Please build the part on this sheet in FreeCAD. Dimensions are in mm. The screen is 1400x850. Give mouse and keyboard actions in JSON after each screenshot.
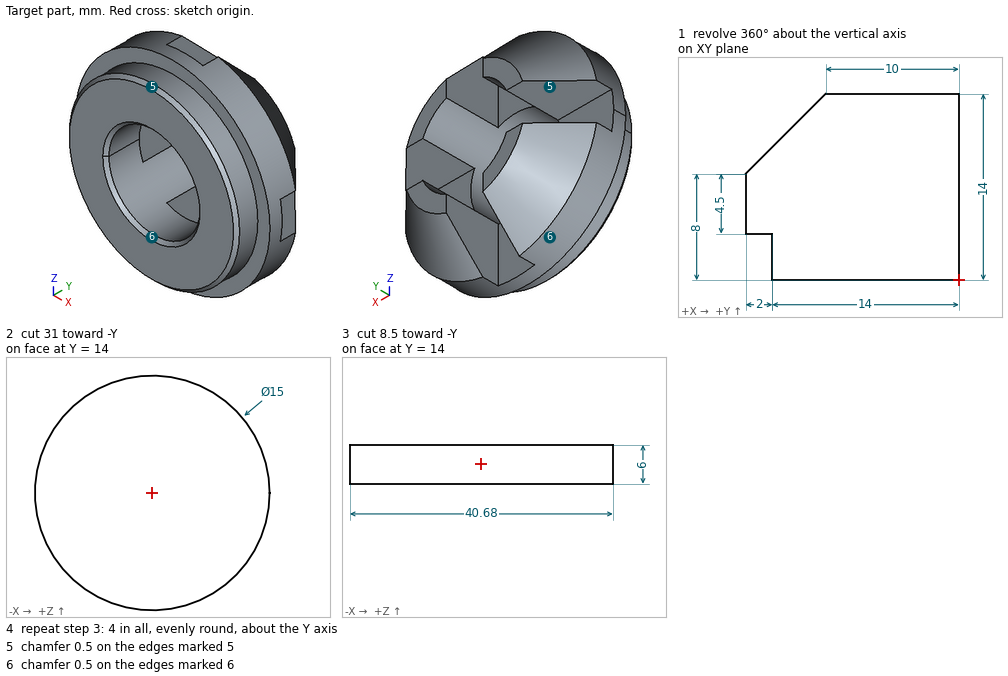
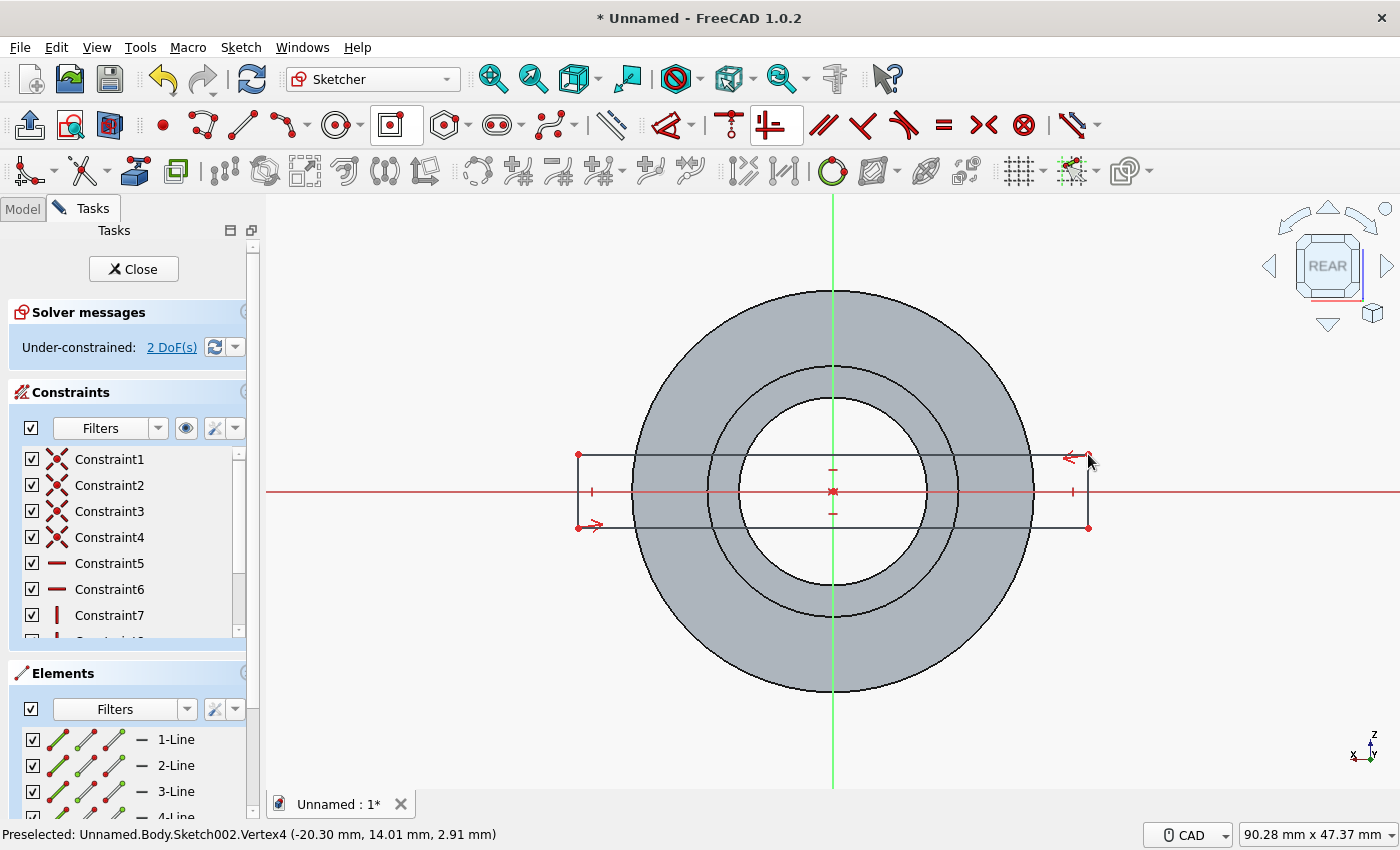
{"action": "left_click", "coordinate": [666, 126]}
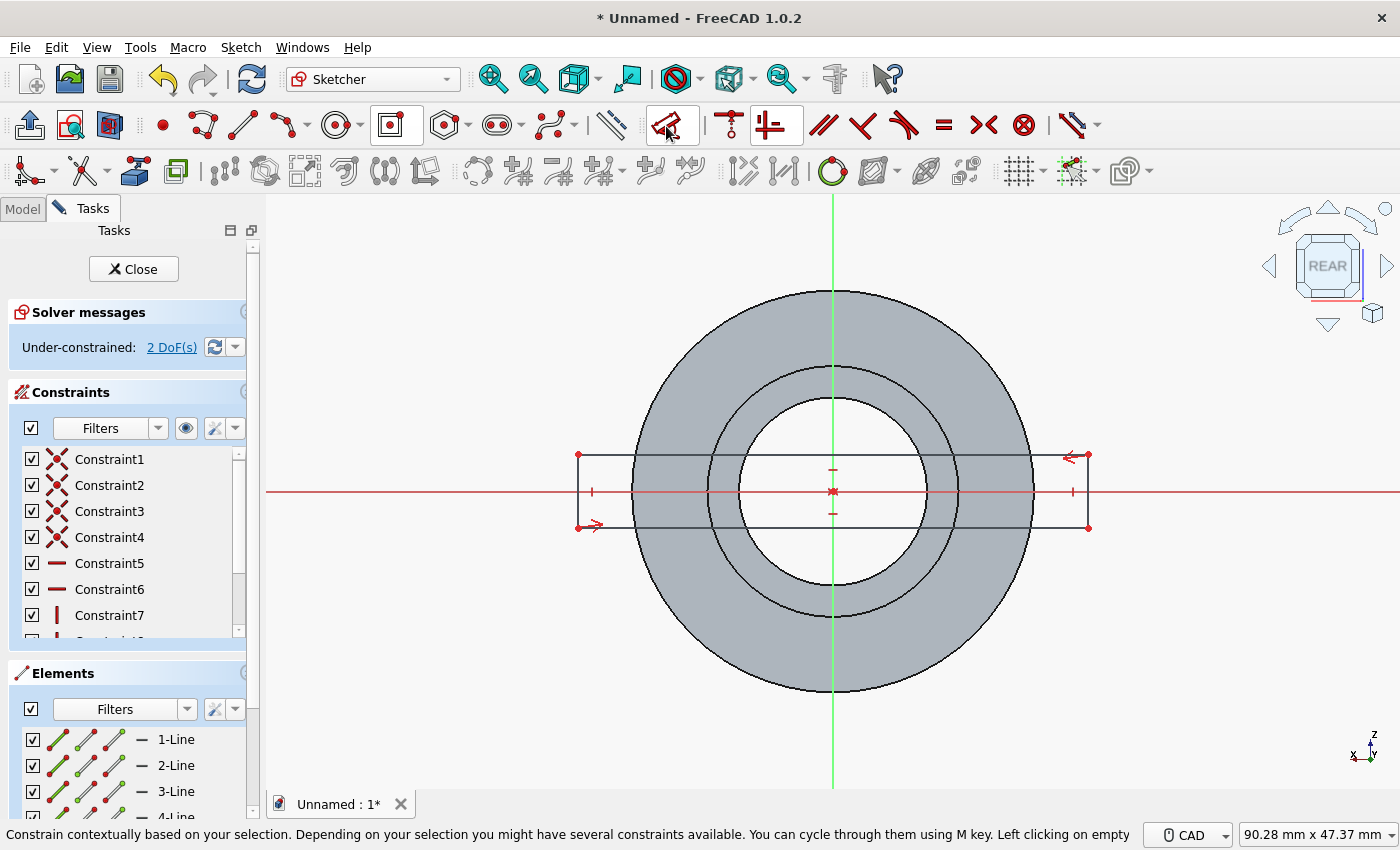
{"action": "left_click", "coordinate": [1088, 506]}
{"action": "left_click", "coordinate": [1122, 475]}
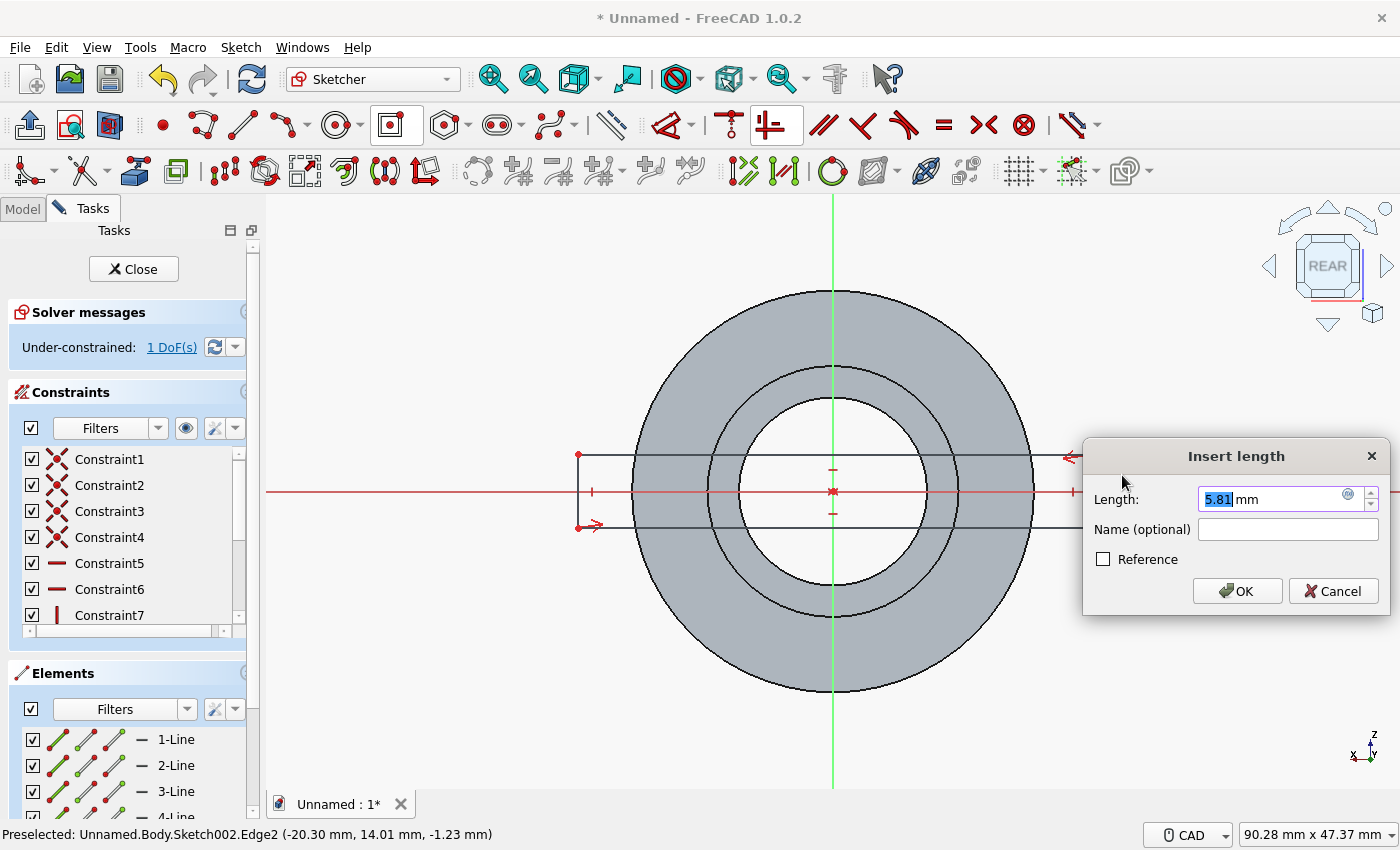
{"action": "type", "text": "6"}
{"action": "key", "text": "Return"}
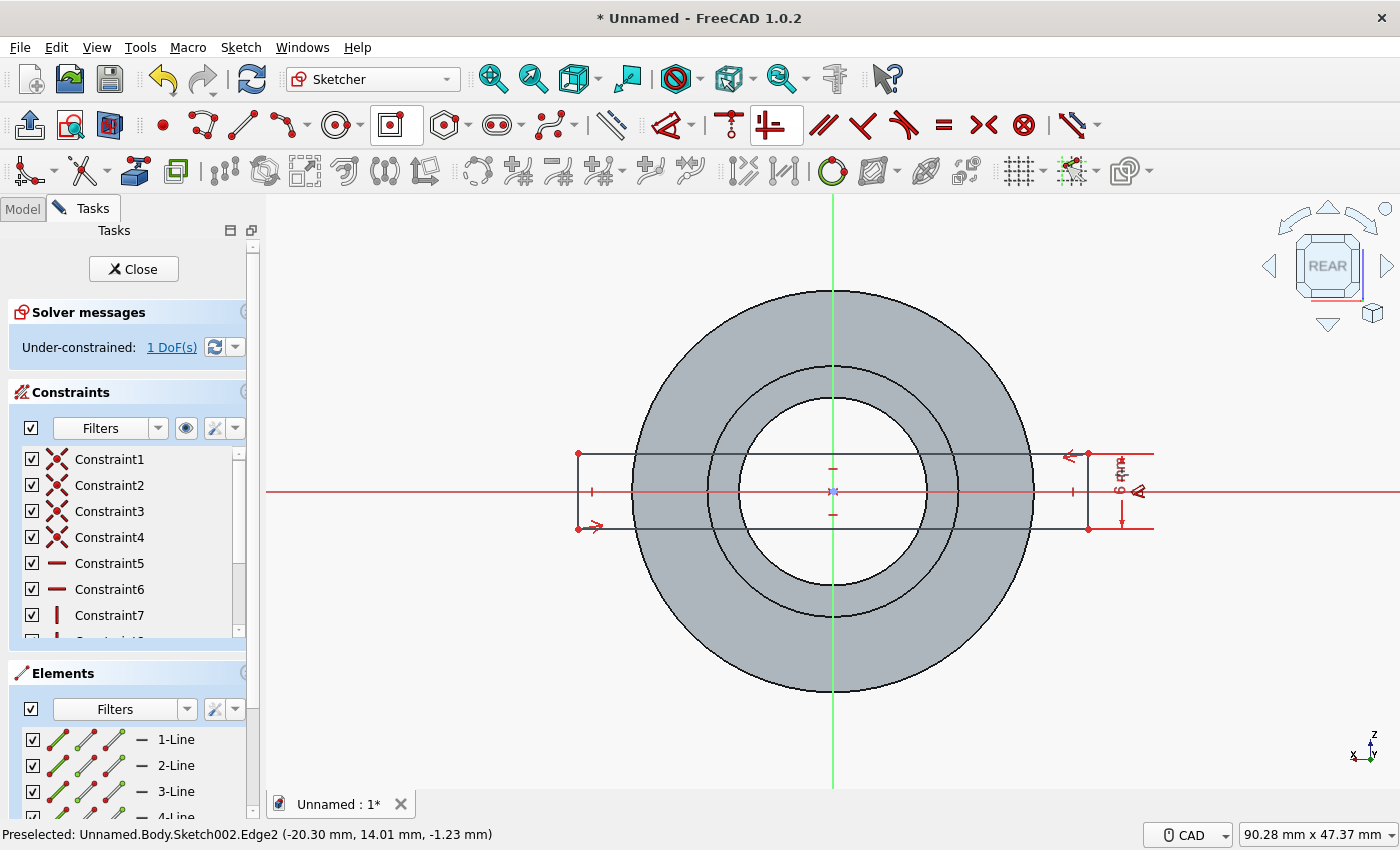
{"action": "left_click", "coordinate": [731, 529]}
{"action": "left_click", "coordinate": [716, 563]}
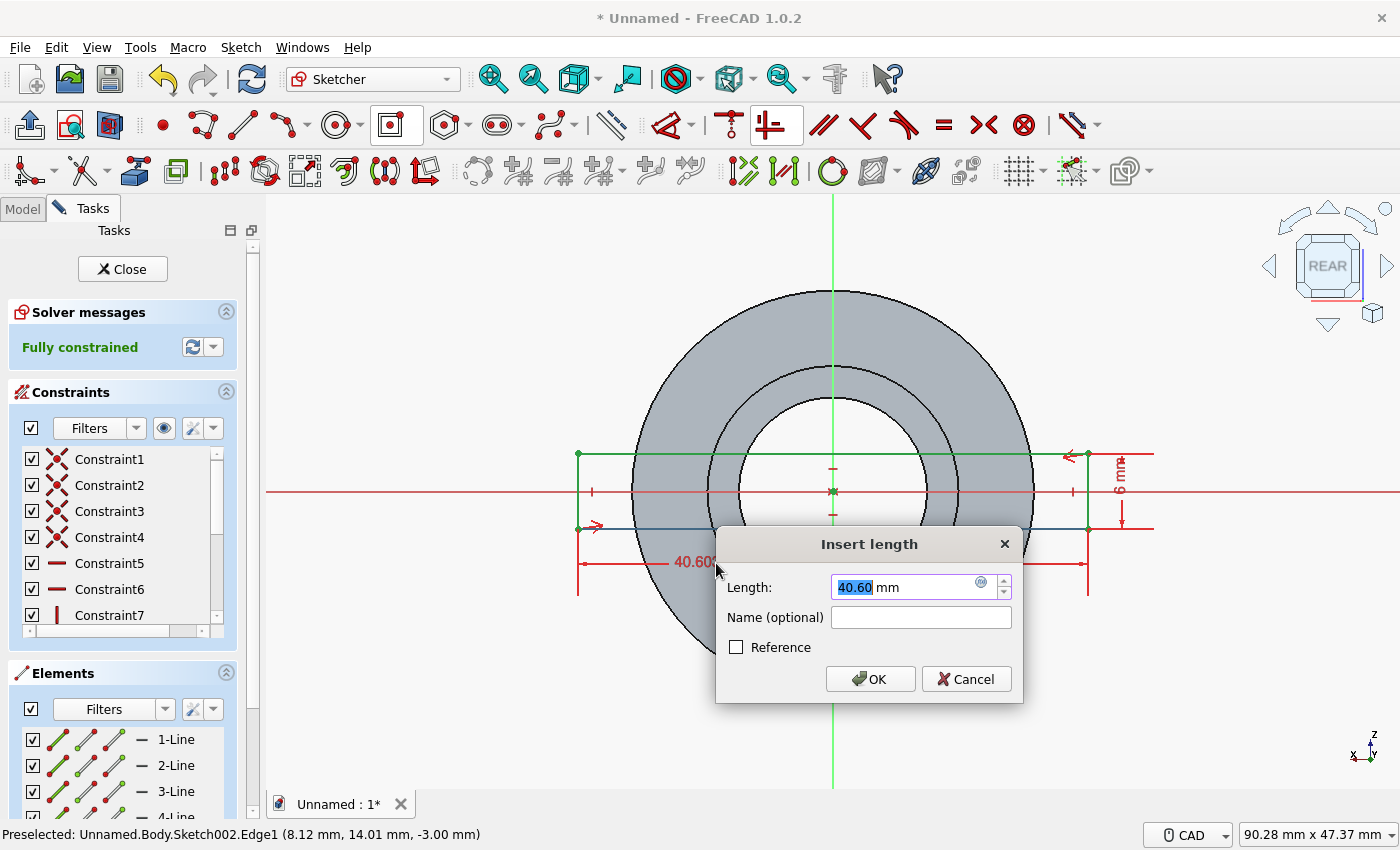
{"action": "type", "text": "40.68"}
{"action": "key", "text": "Return"}
{"action": "key", "text": "Escape"}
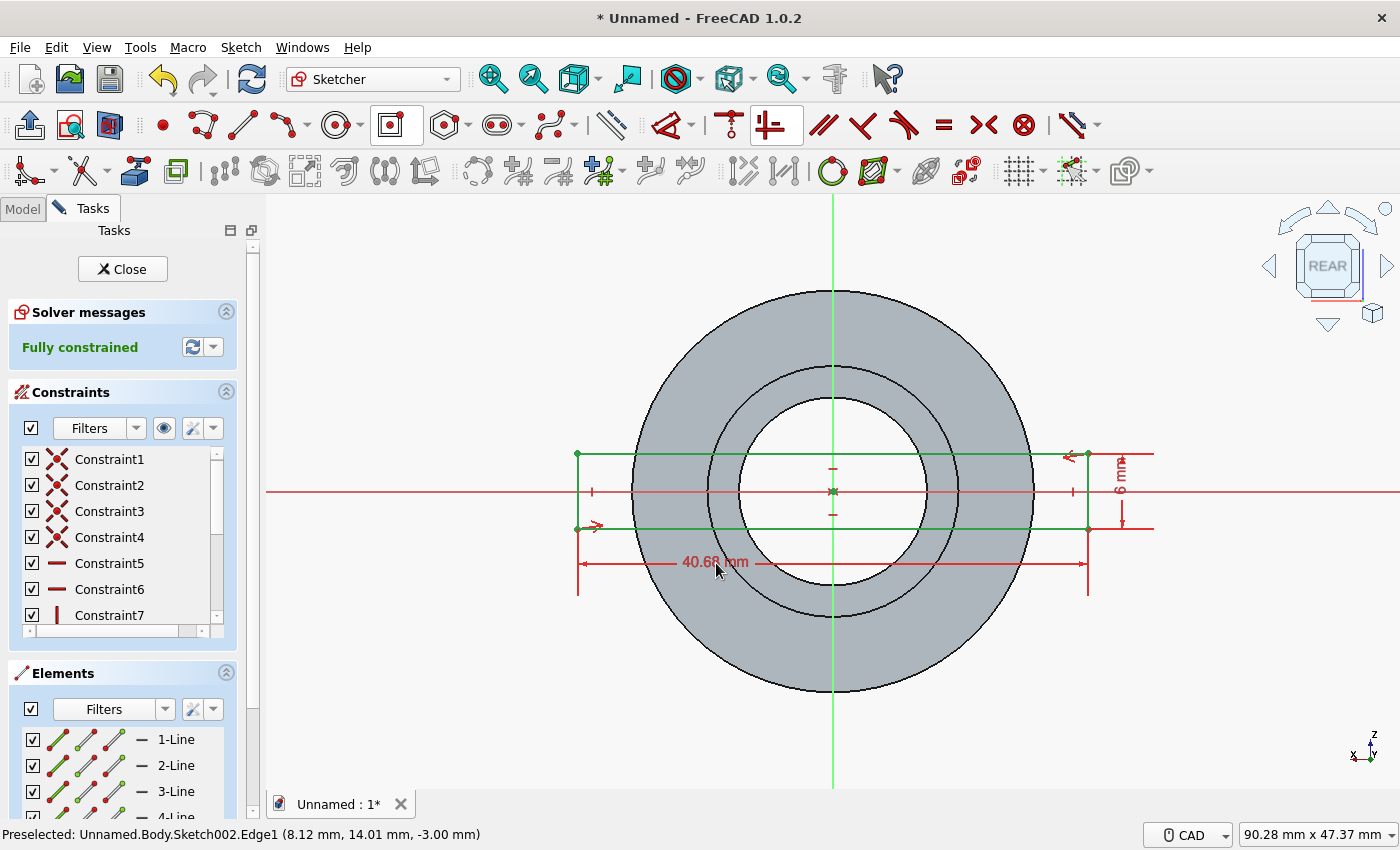
{"action": "left_click", "coordinate": [123, 269]}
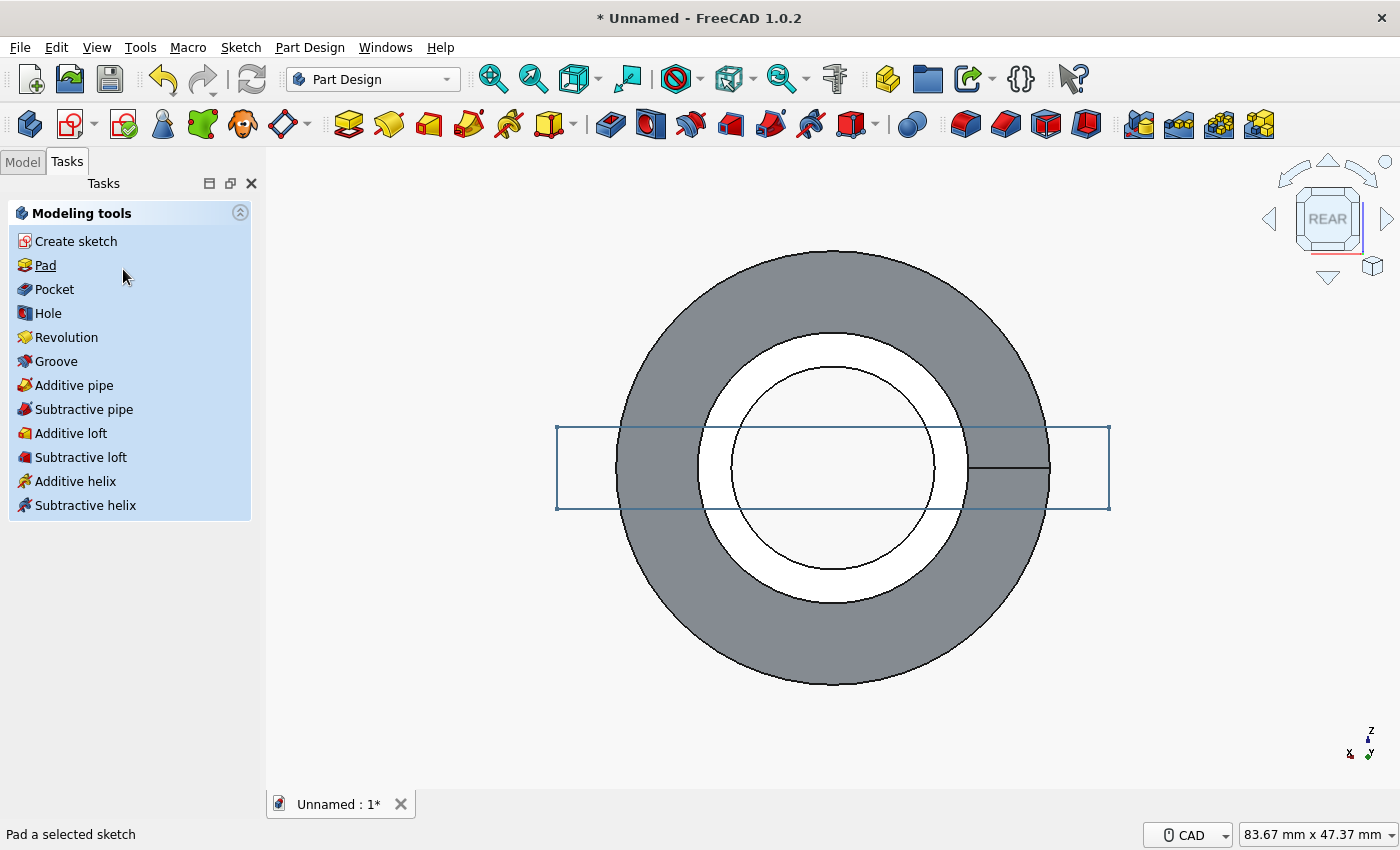
{"action": "left_click", "coordinate": [612, 124]}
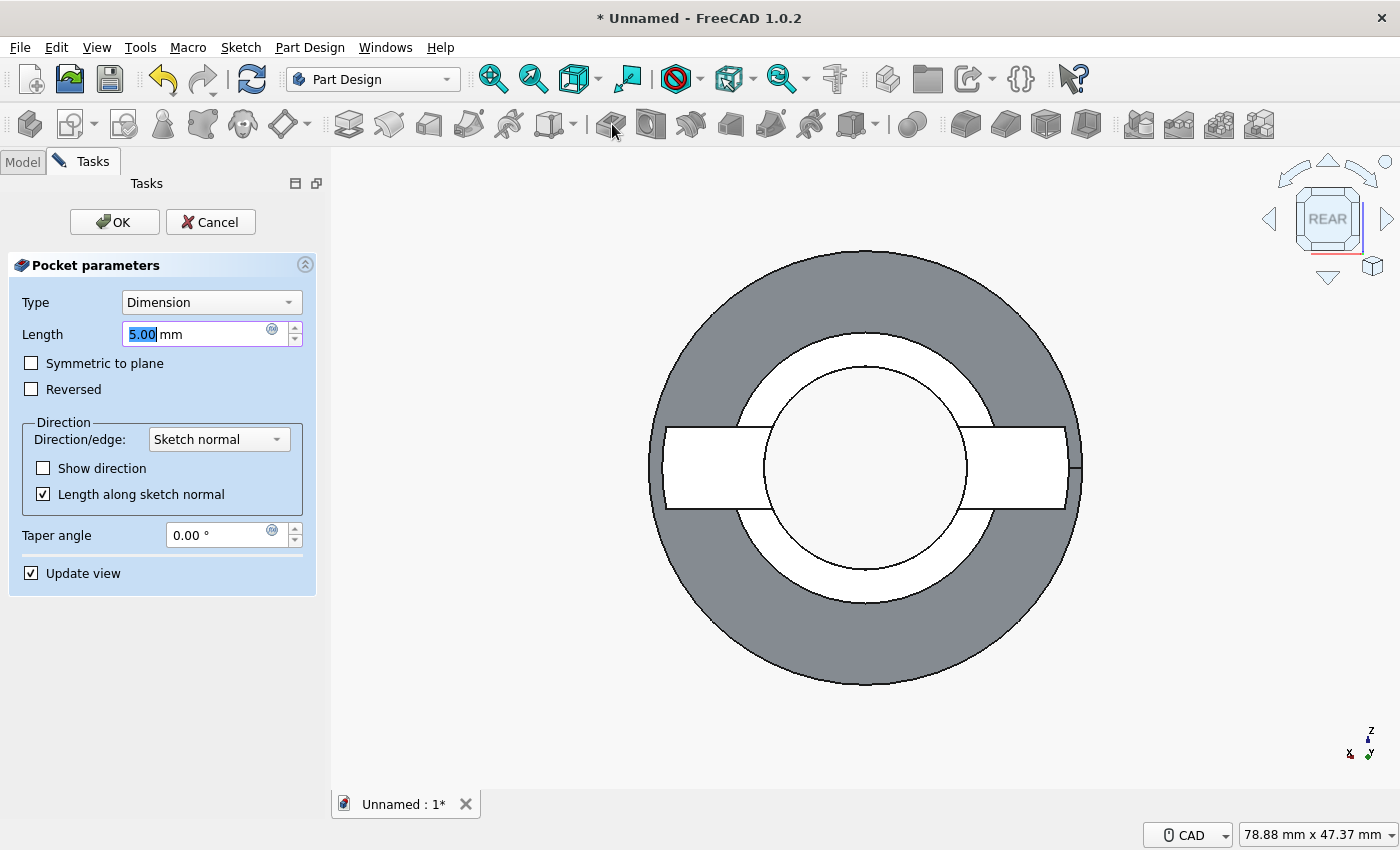
{"action": "type", "text": "8.5"}
{"action": "key", "text": "Tab"}